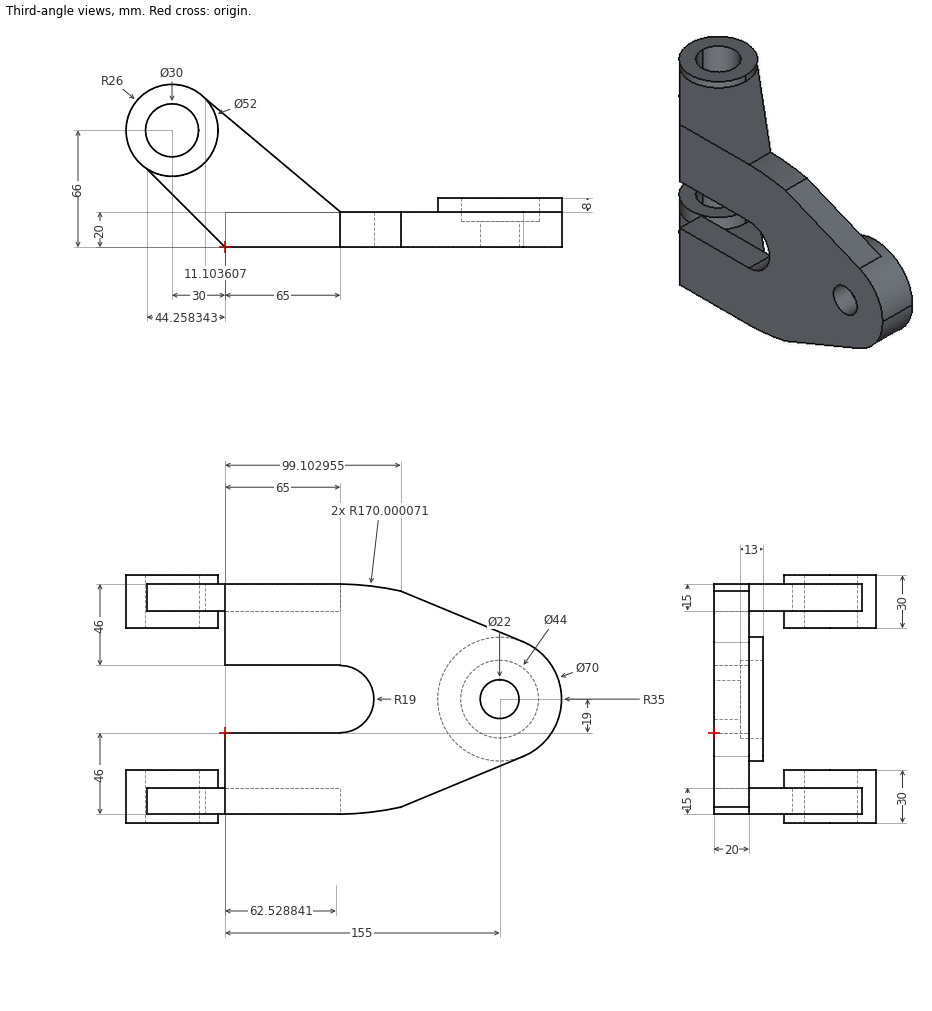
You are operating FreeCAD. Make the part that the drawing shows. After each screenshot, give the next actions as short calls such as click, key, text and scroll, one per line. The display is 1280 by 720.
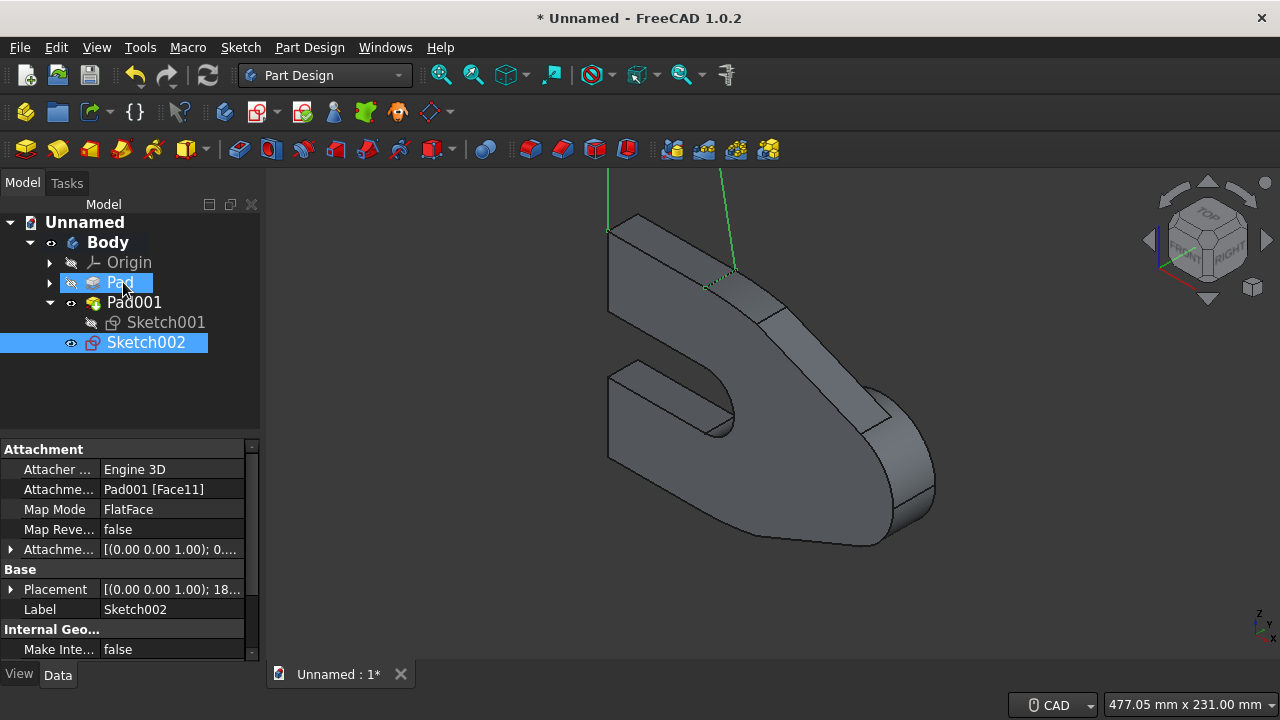
click(26, 150)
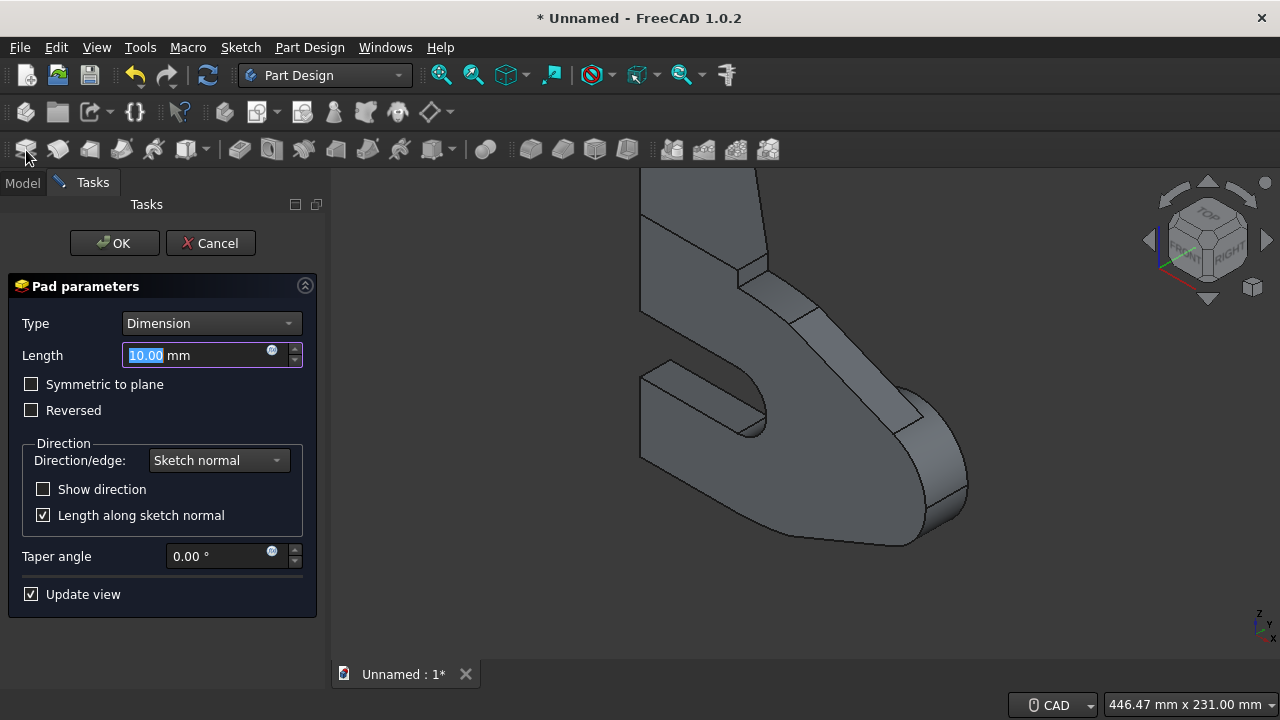
text(15)
key(Tab)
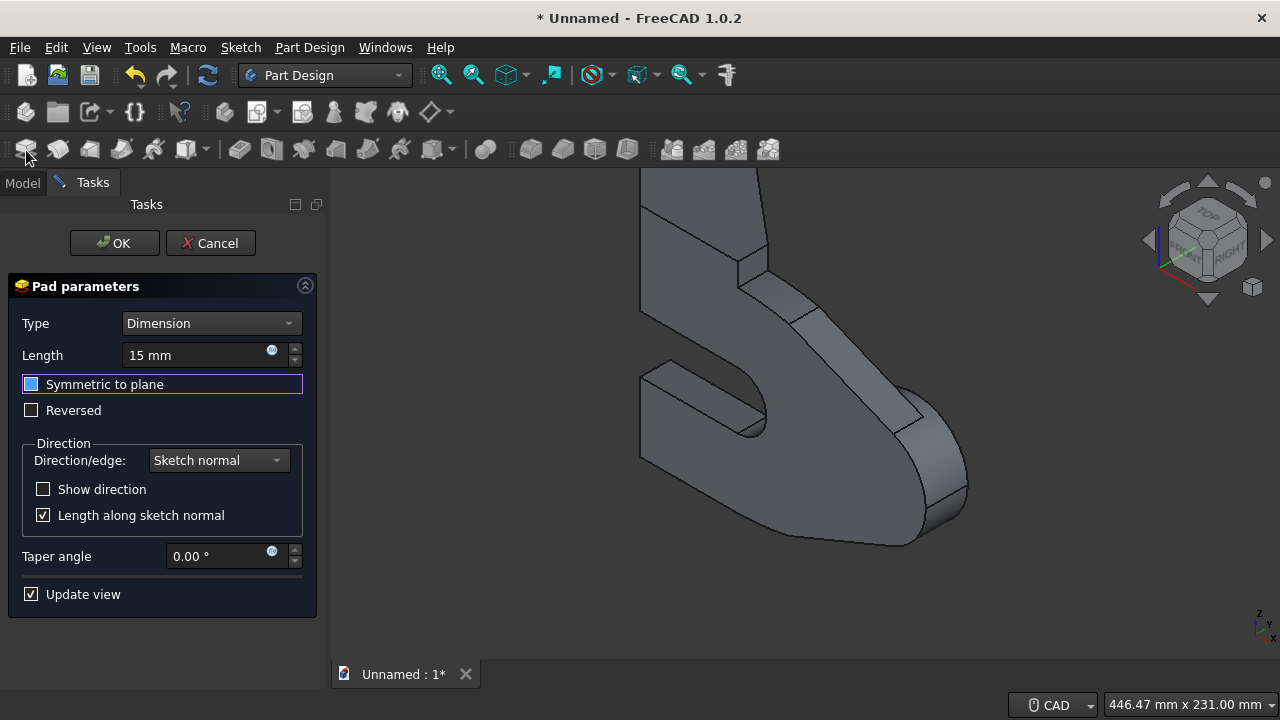
click(30, 410)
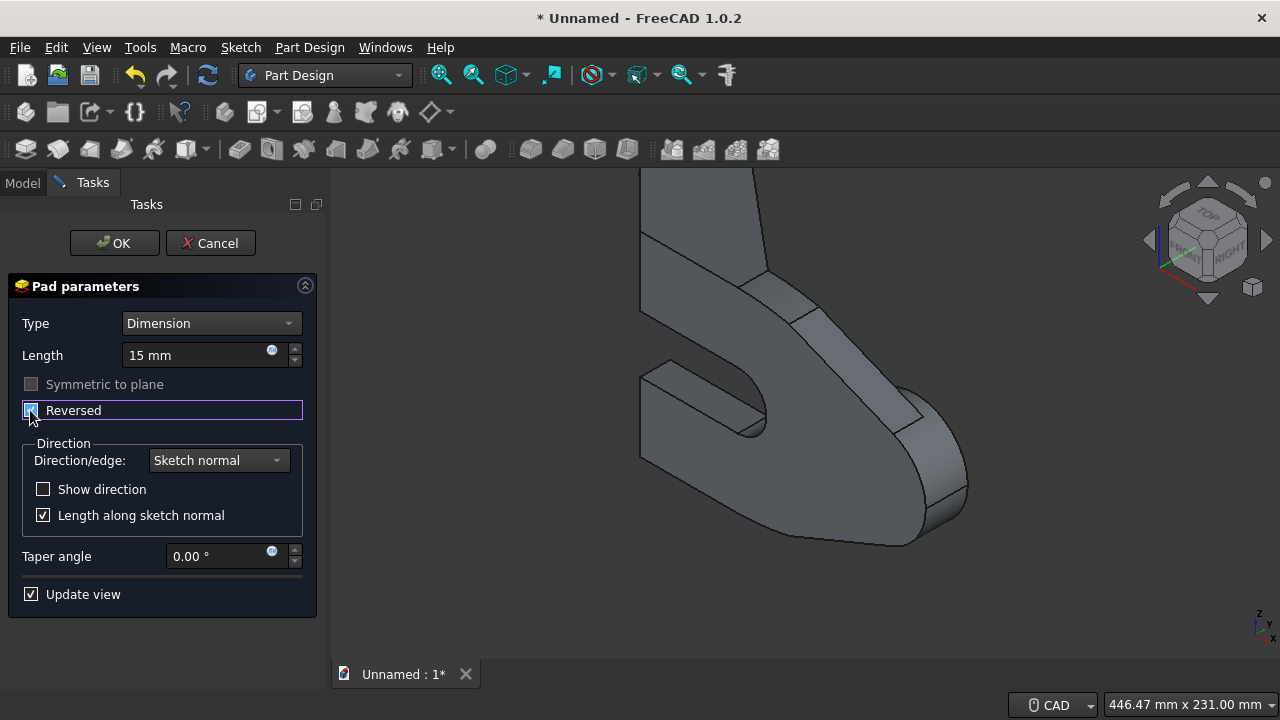
click(115, 243)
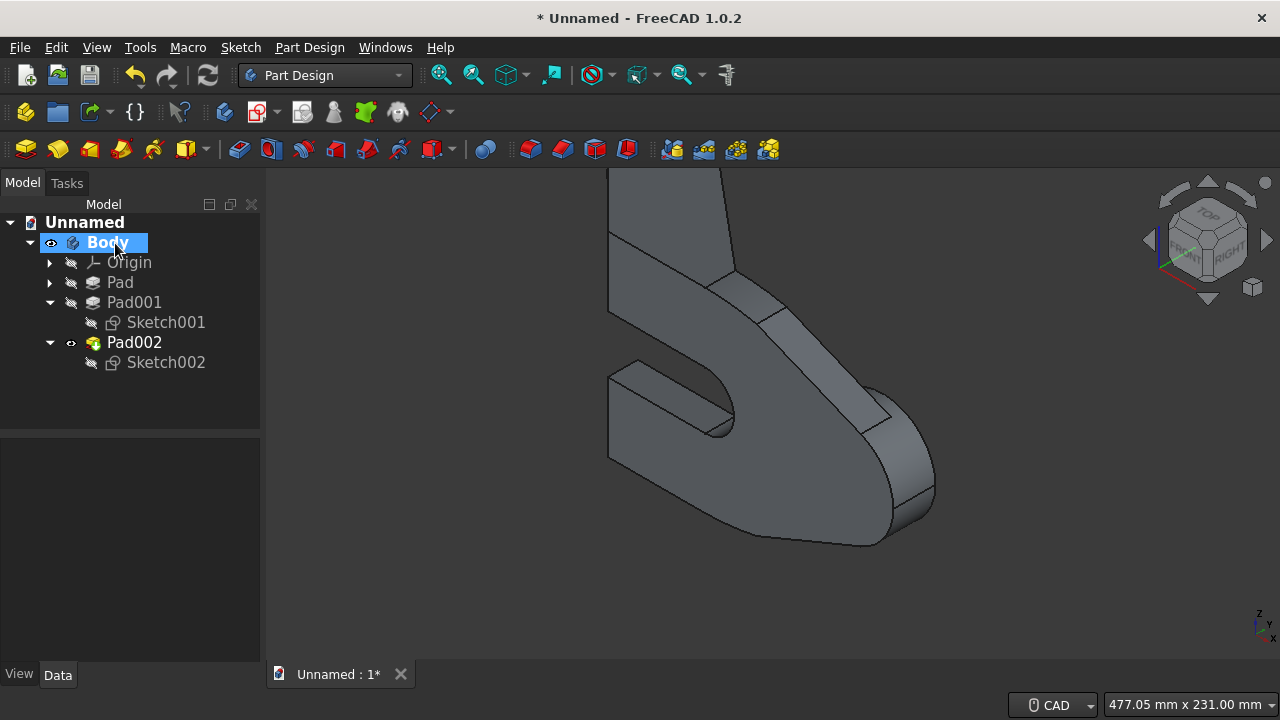
key(v)
key(f)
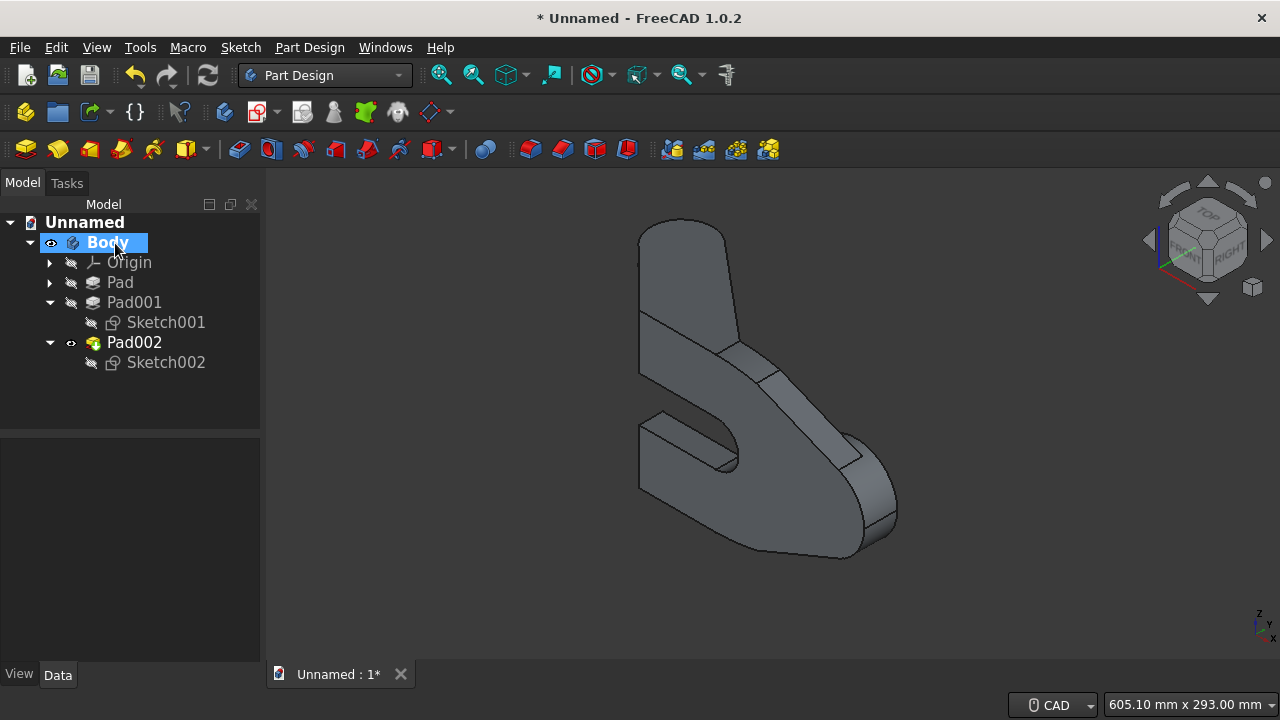
click(50, 263)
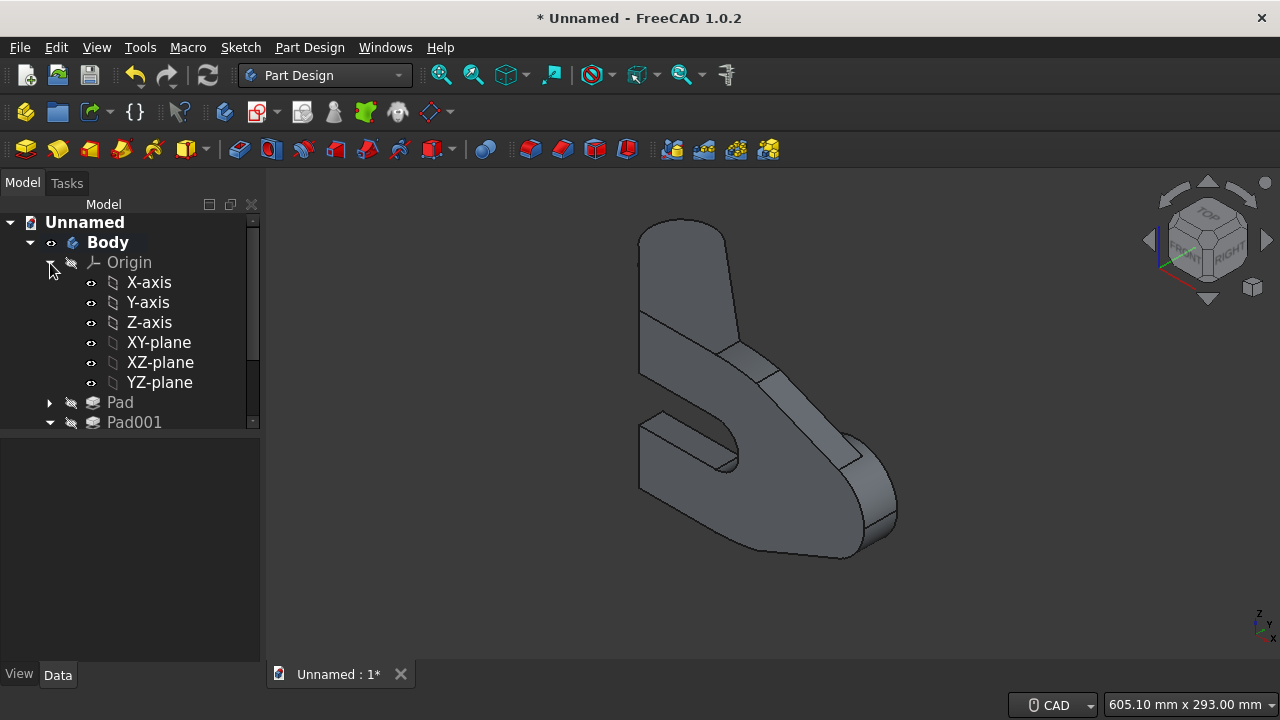
click(136, 343)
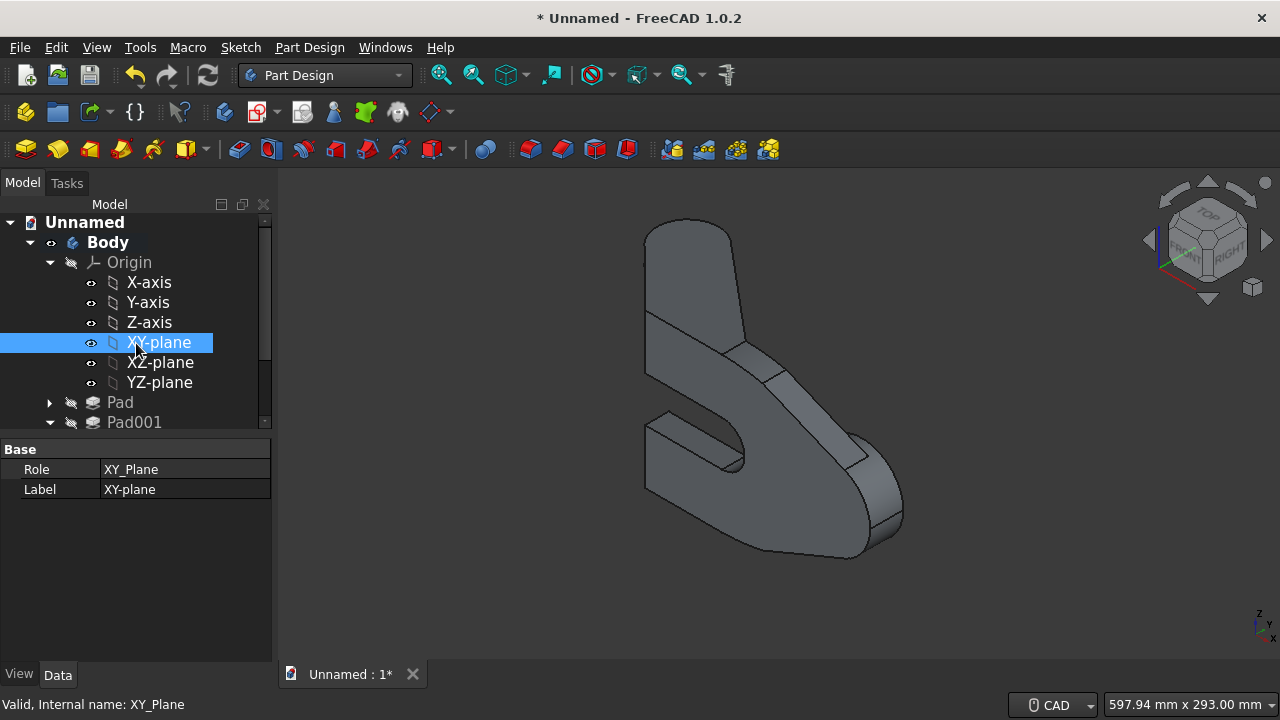
click(430, 112)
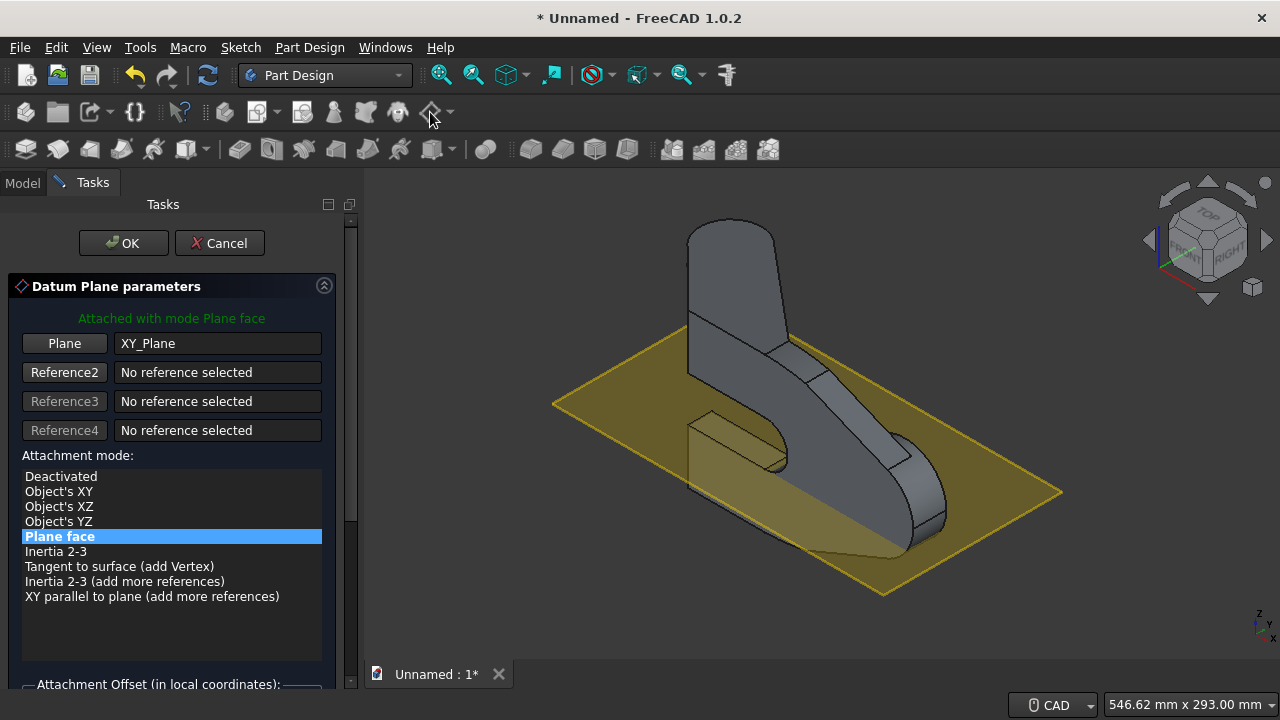
scroll(351, 451, down, 3)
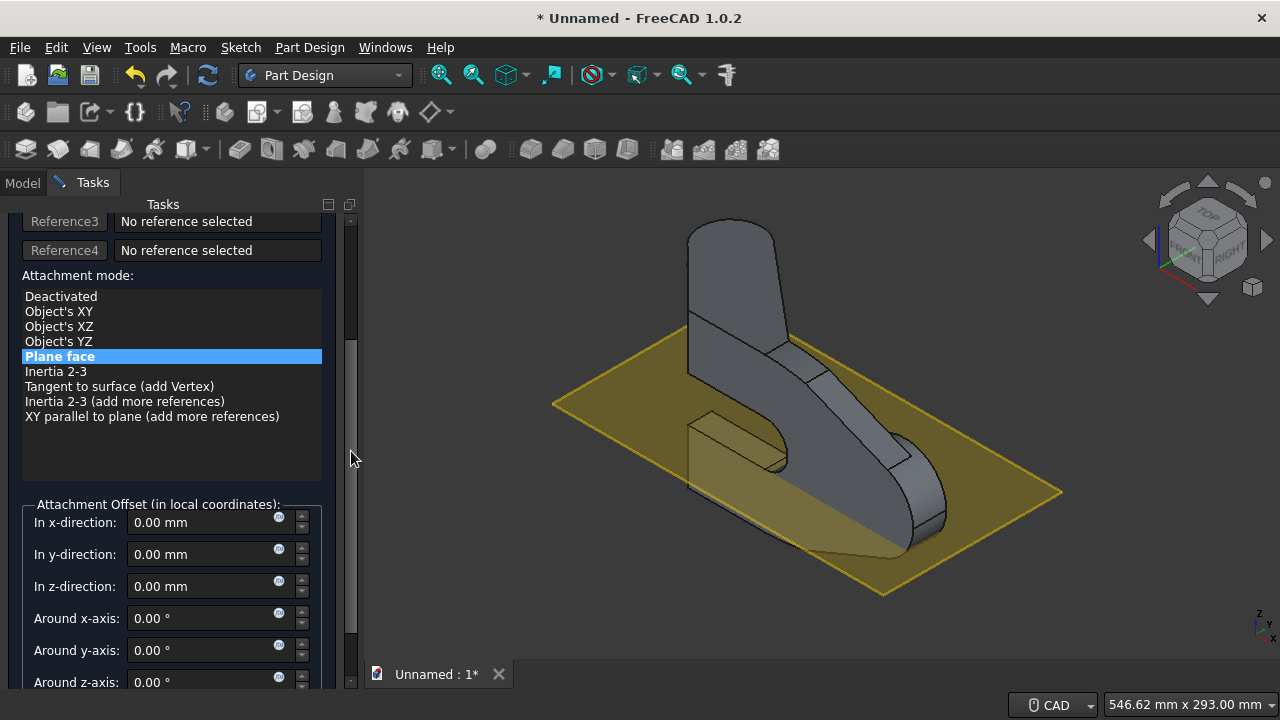
triple_click(210, 586)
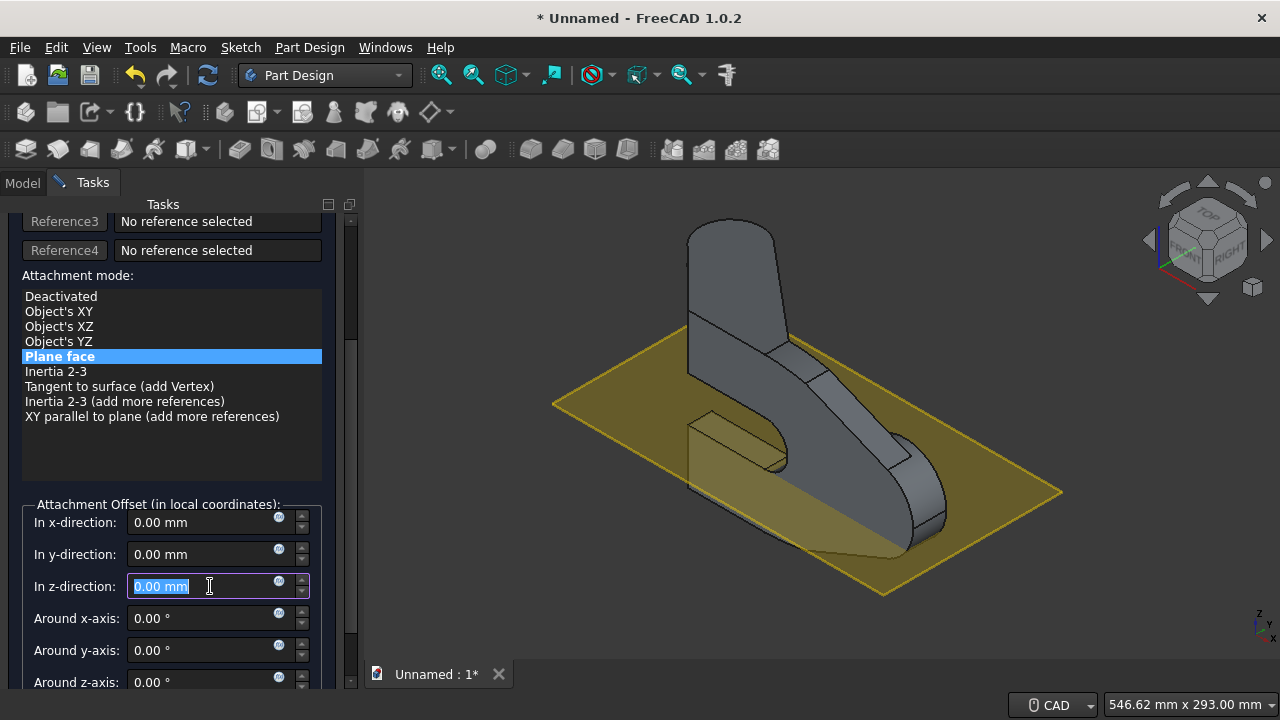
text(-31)
key(Tab)